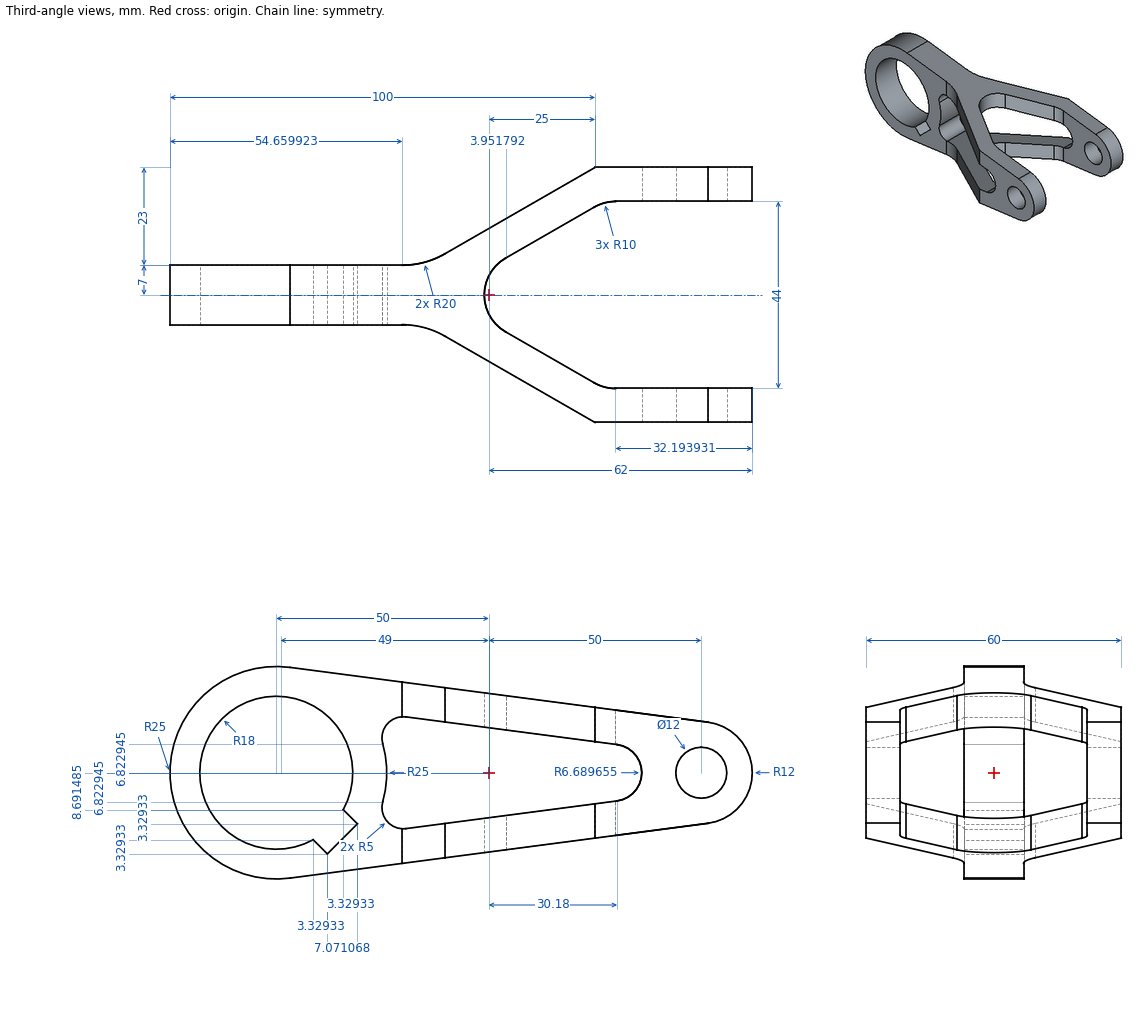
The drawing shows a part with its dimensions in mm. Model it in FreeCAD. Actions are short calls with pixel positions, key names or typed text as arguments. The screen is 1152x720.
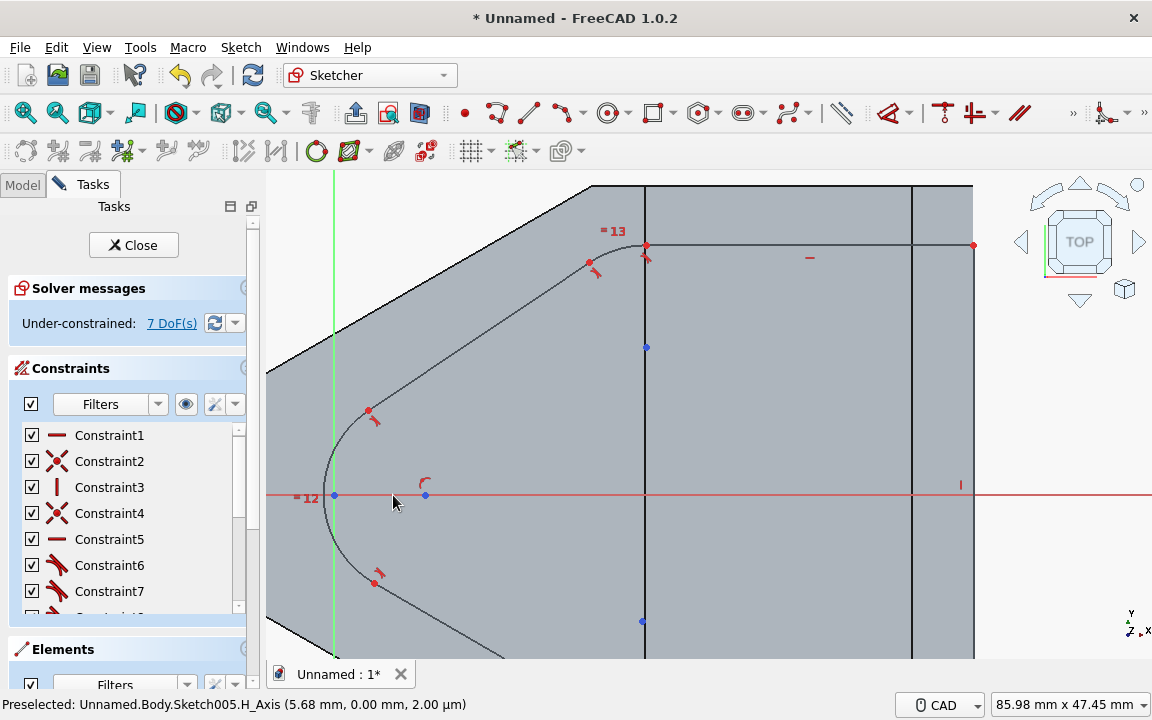
click(643, 621)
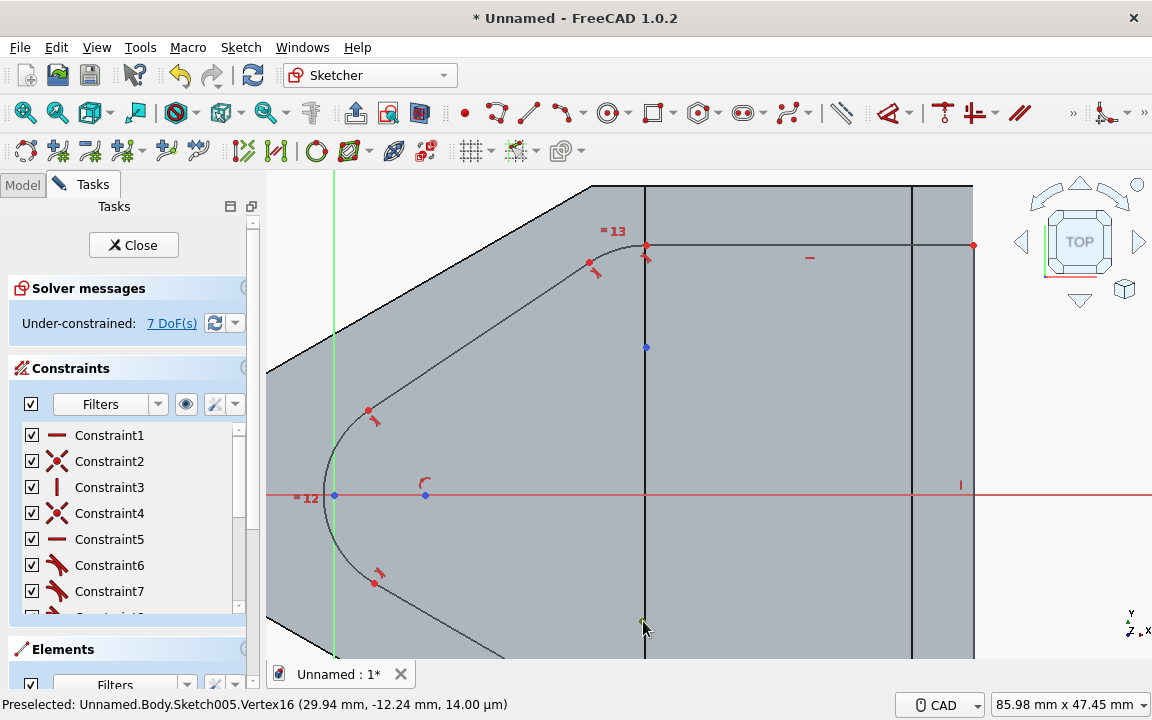
click(646, 347)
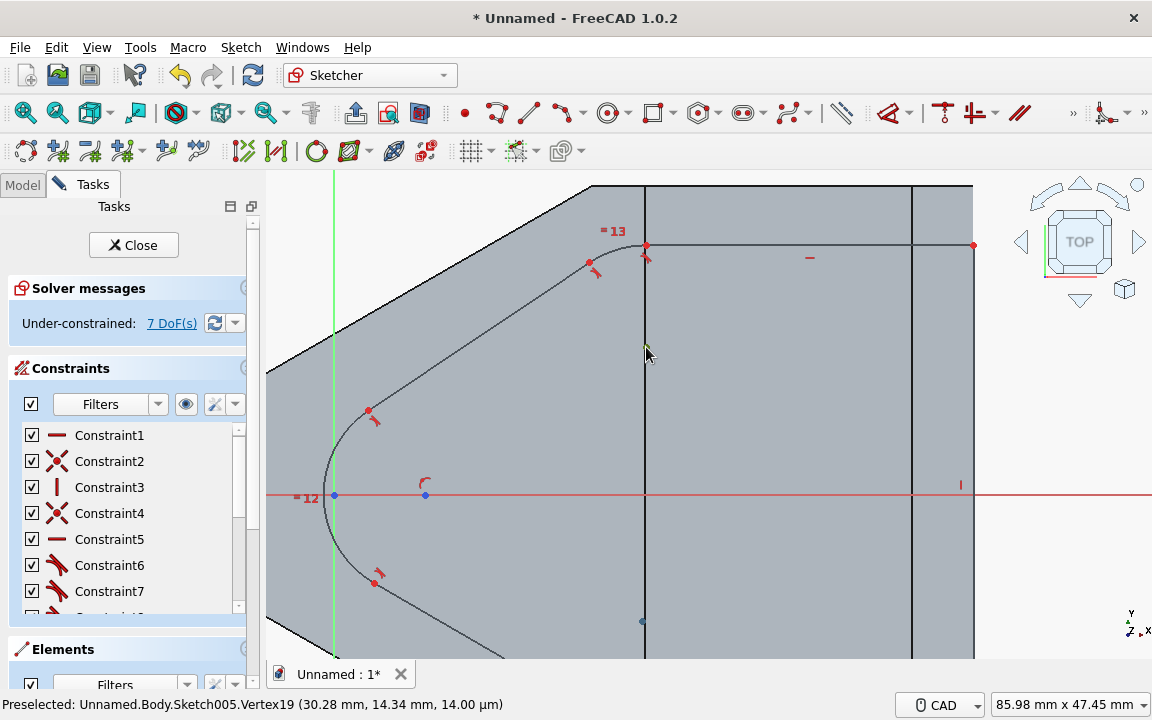
click(393, 495)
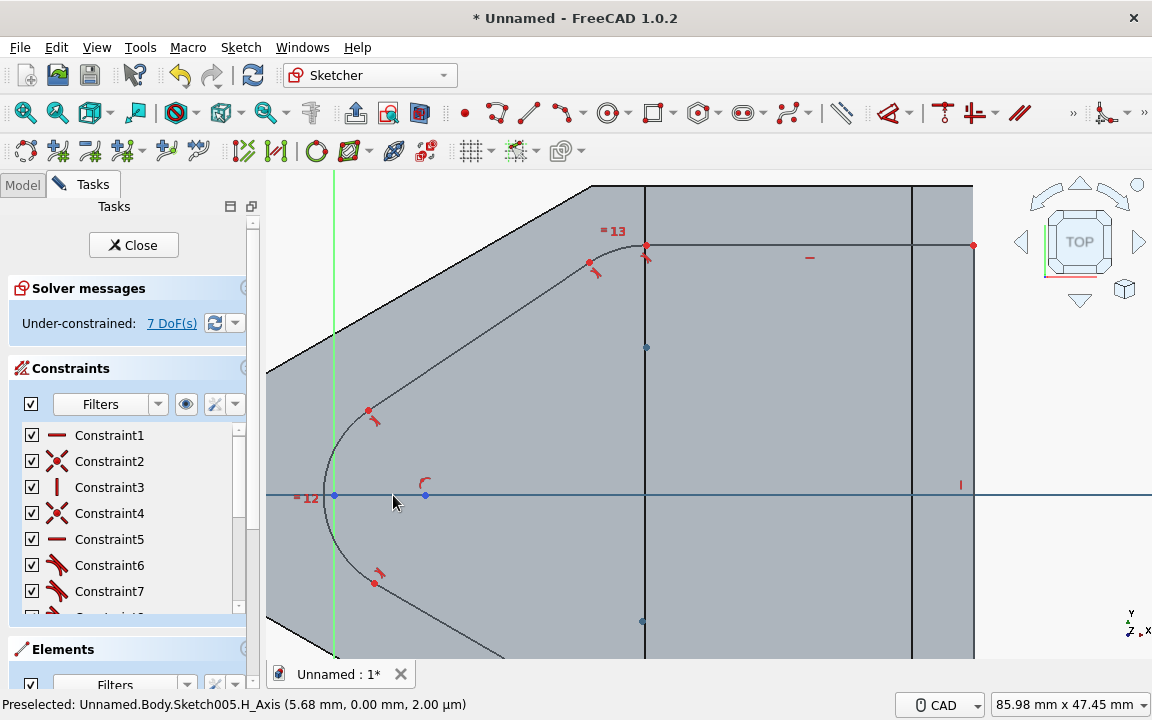
key(s)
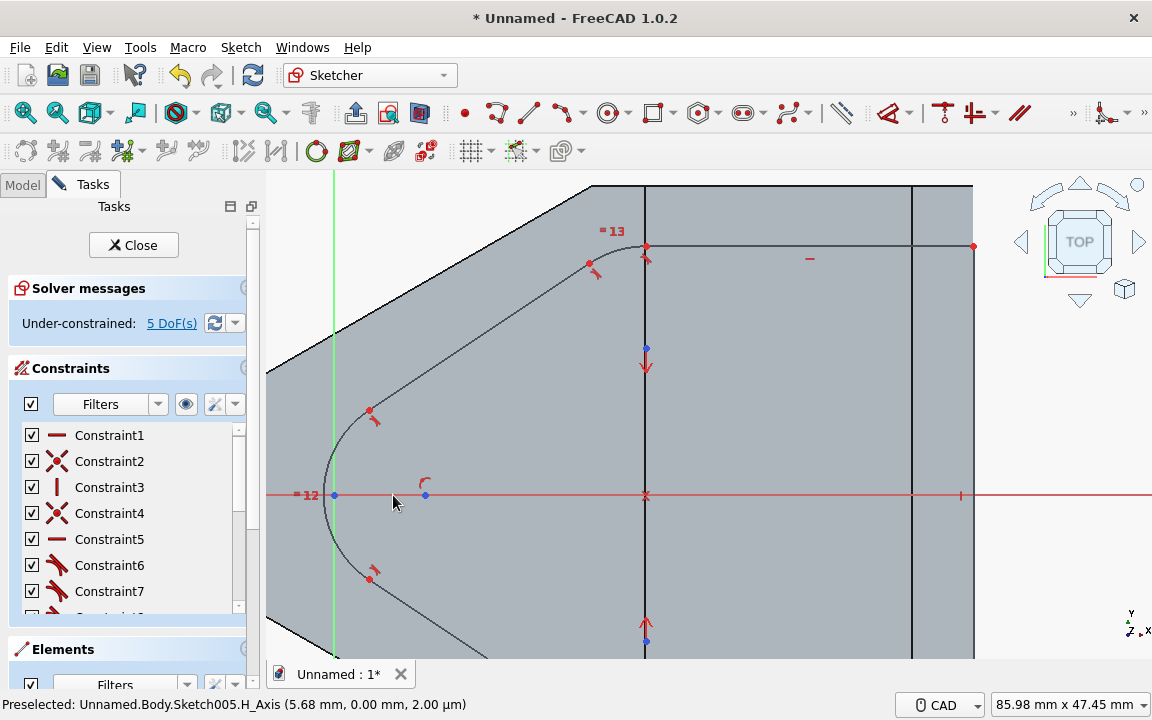
click(888, 114)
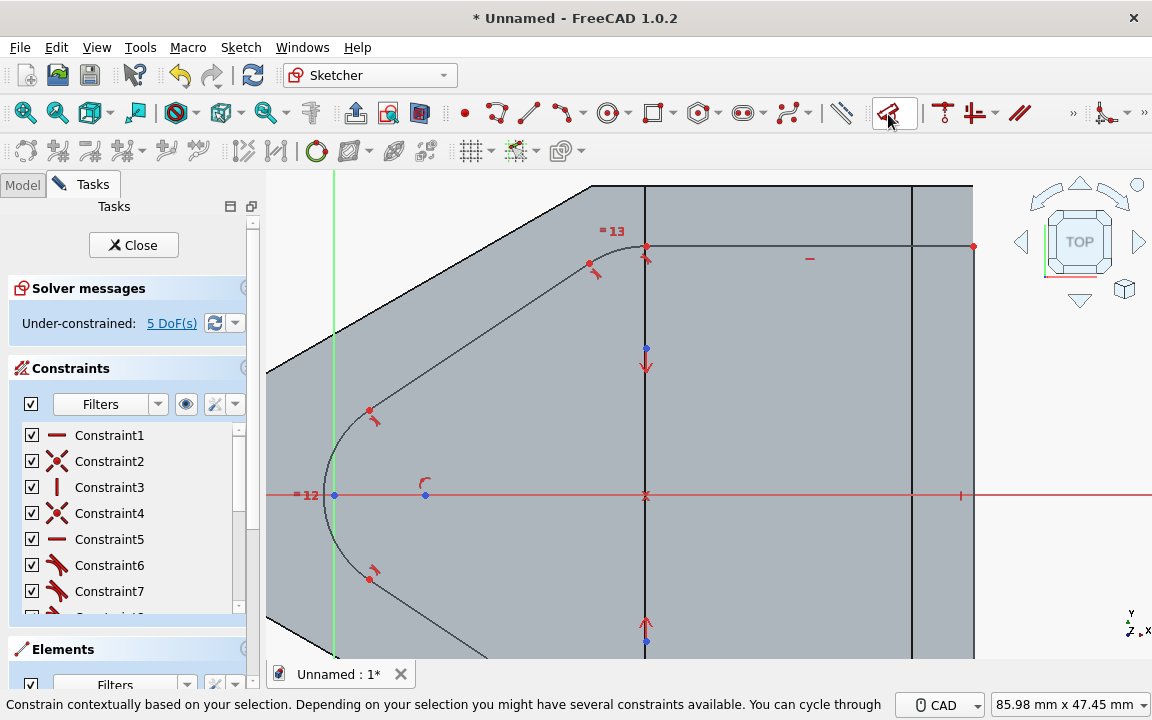
click(332, 456)
click(302, 444)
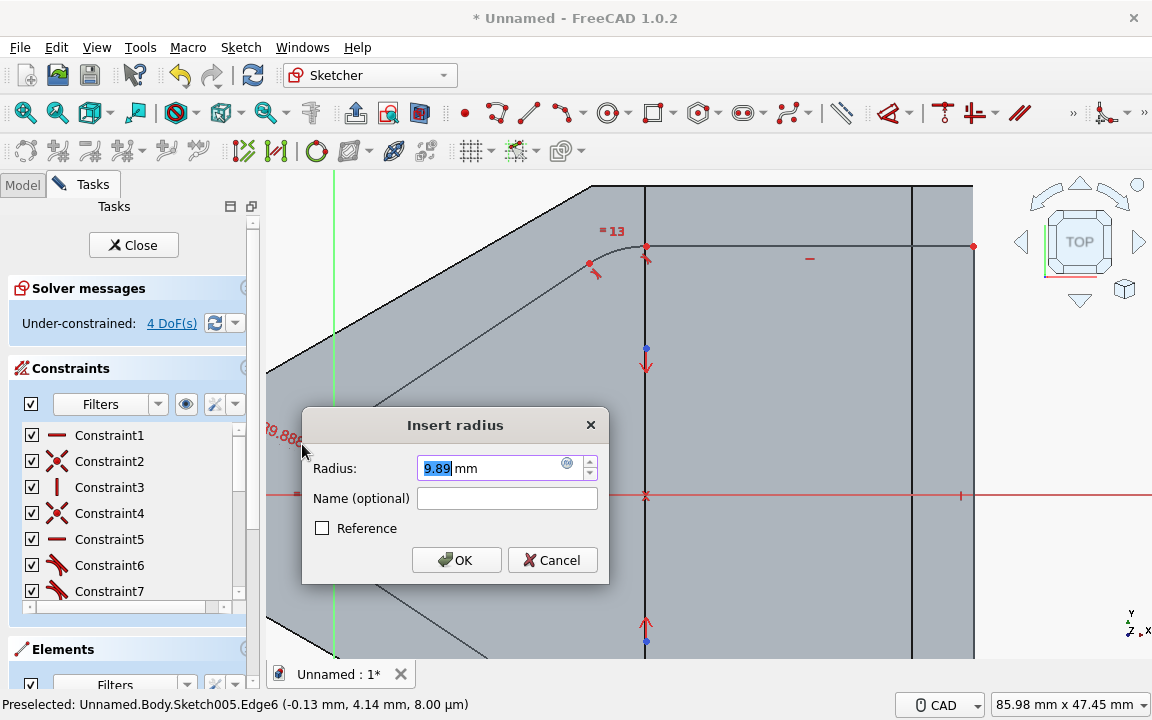
text(10)
key(Return)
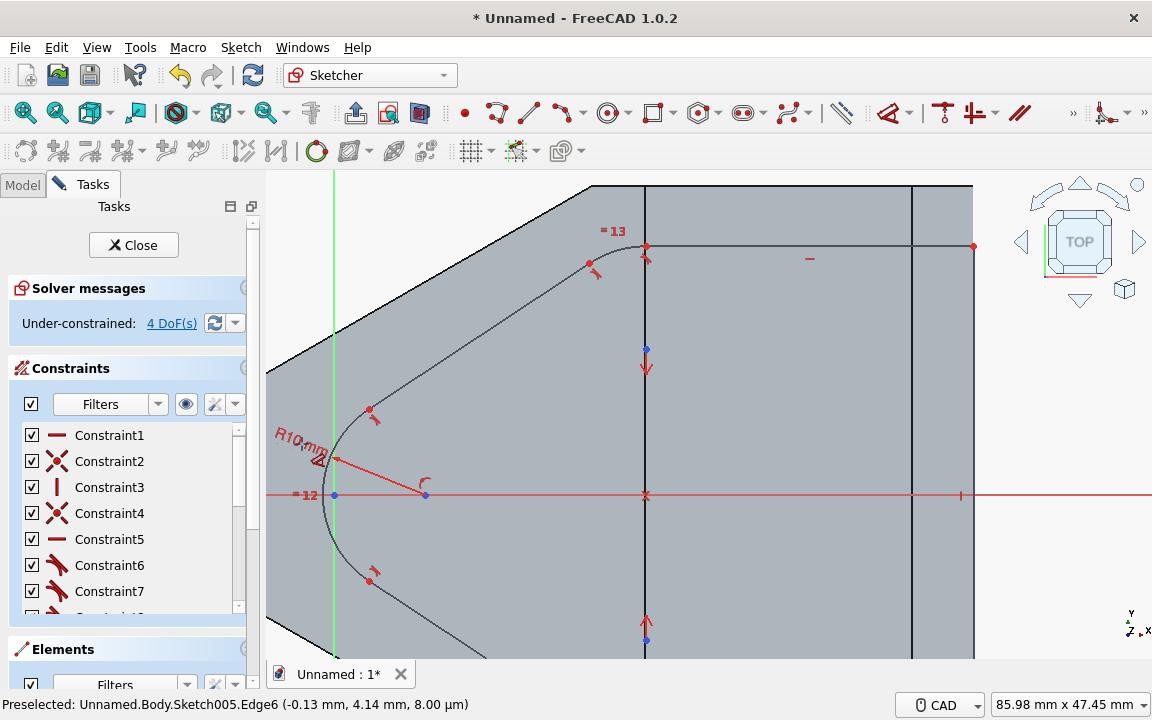
click(974, 595)
click(940, 439)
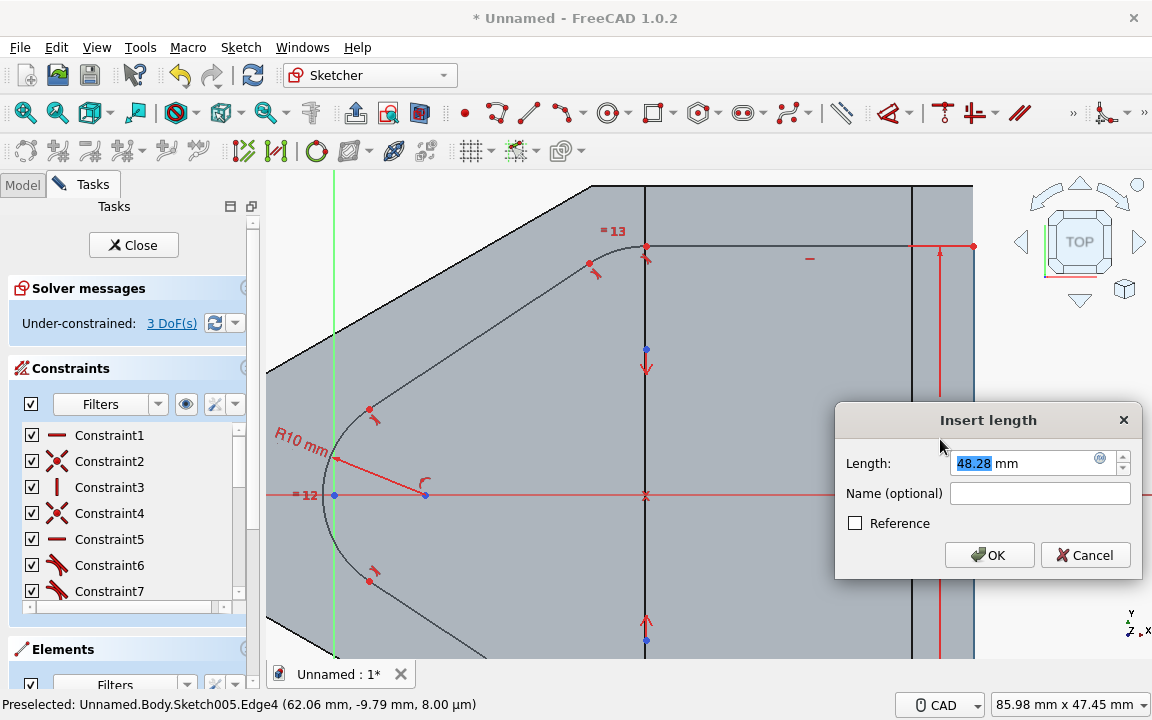
text(44)
key(Return)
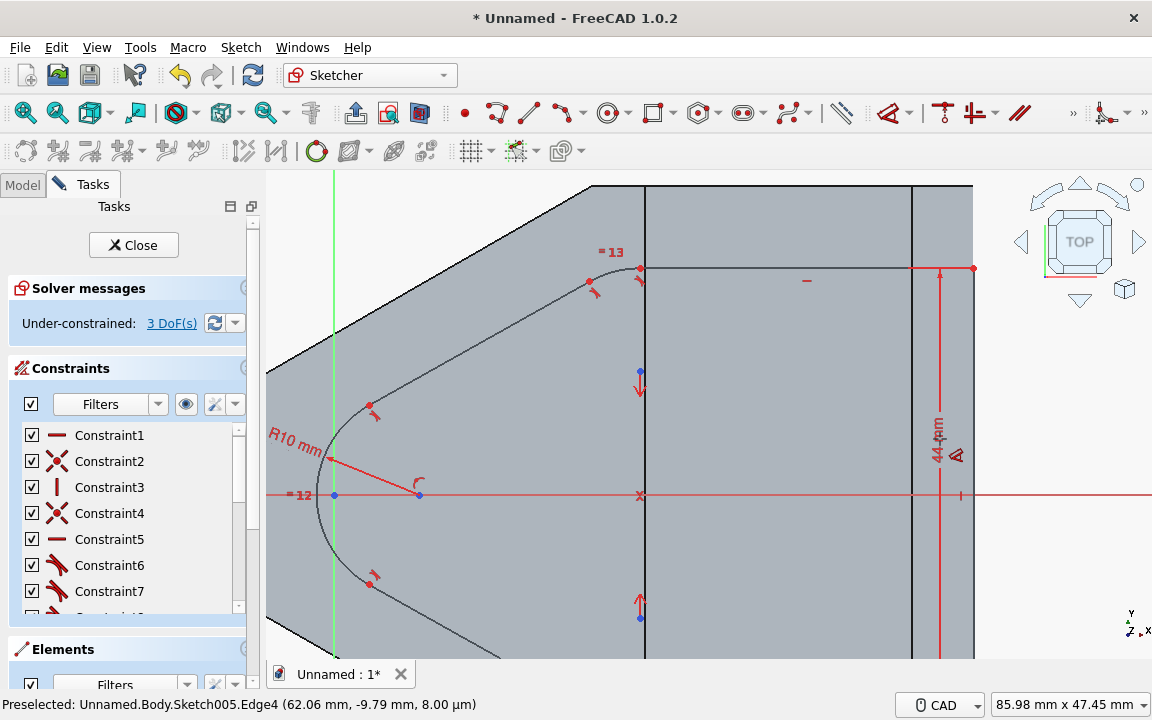
scroll(624, 251, down, 2)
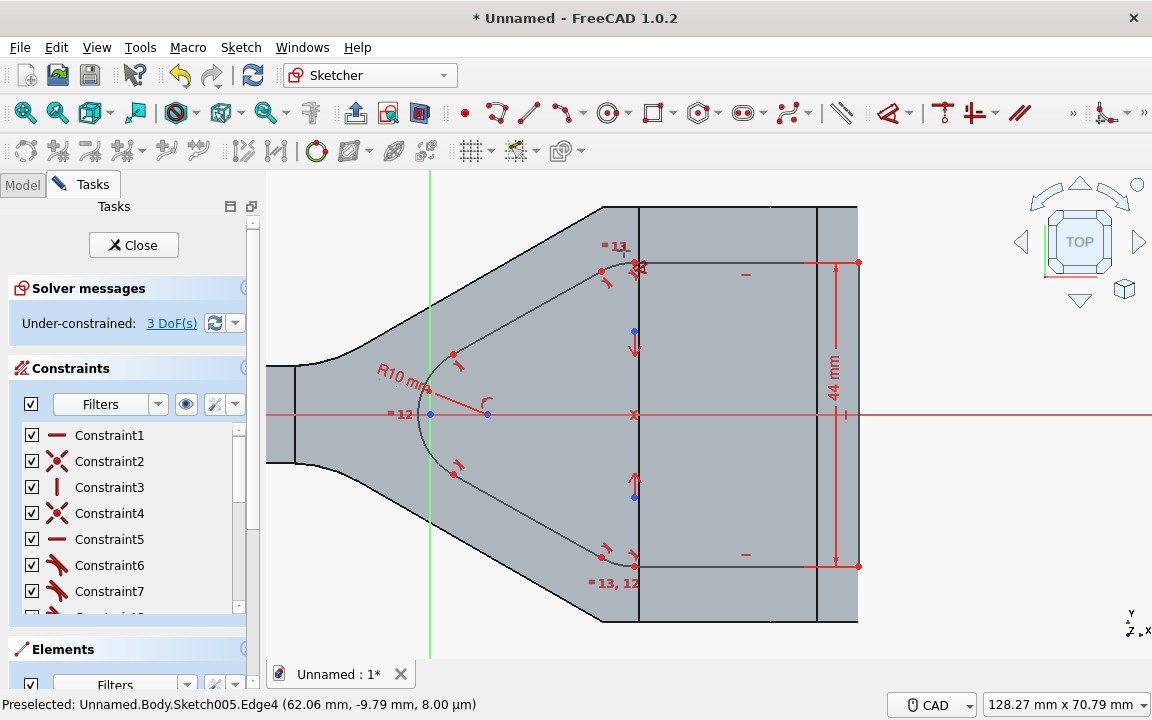
click(859, 567)
click(644, 601)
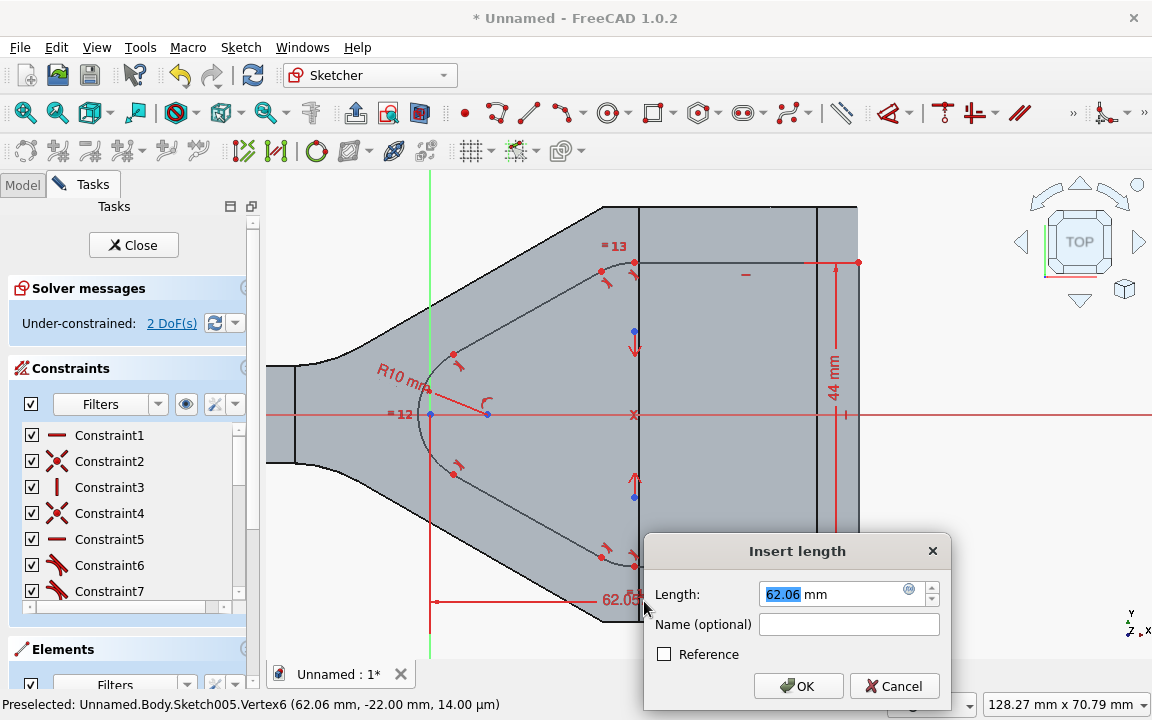
text(62)
key(Return)